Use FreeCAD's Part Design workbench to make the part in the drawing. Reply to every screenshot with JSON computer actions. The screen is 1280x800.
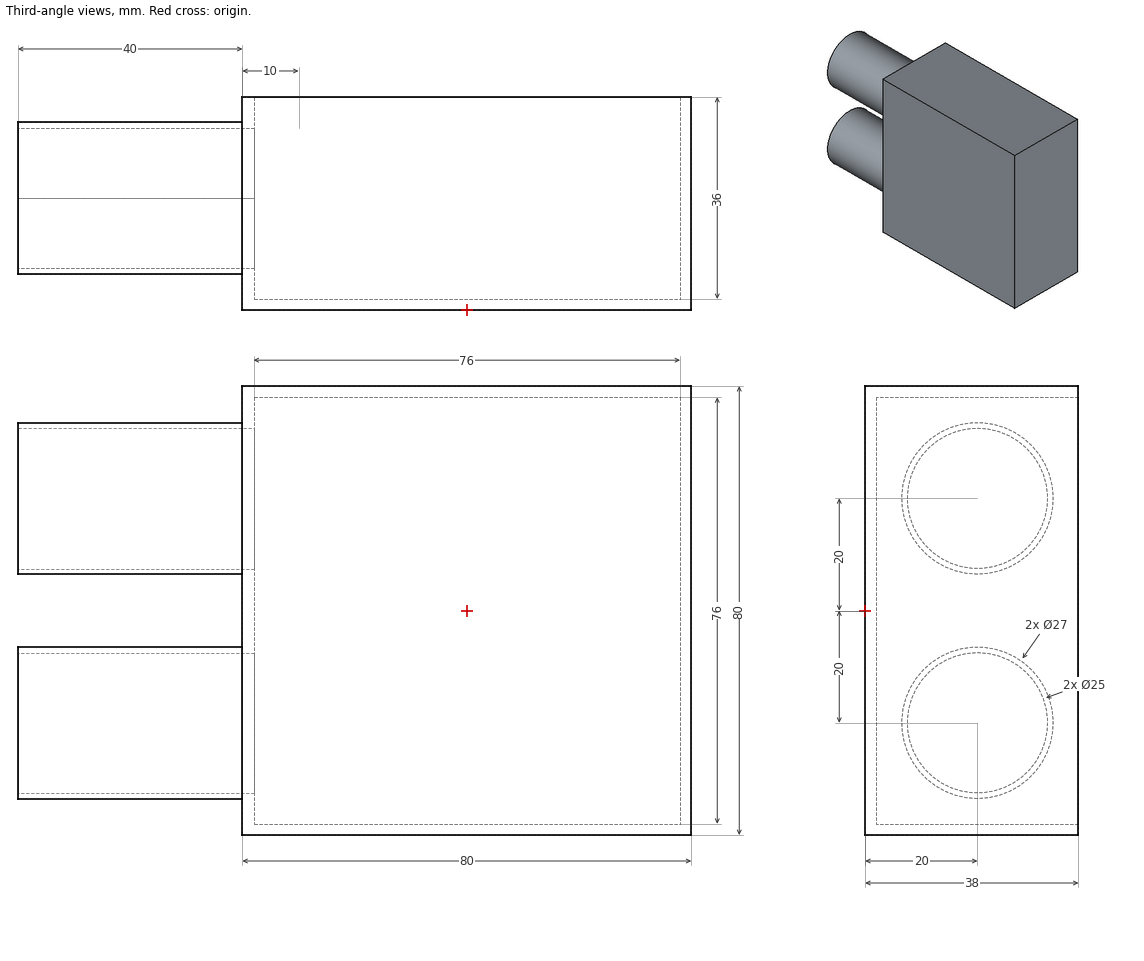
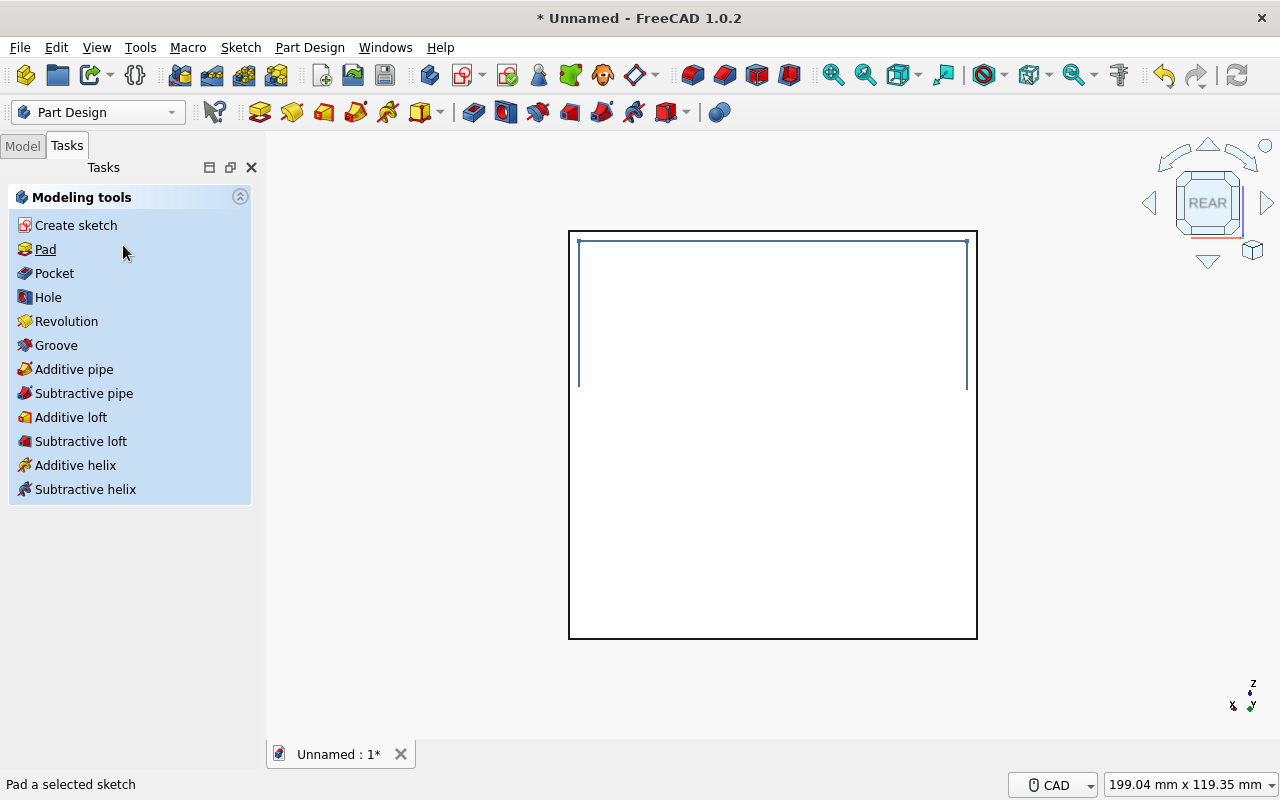
{"action": "left_click", "coordinate": [474, 112]}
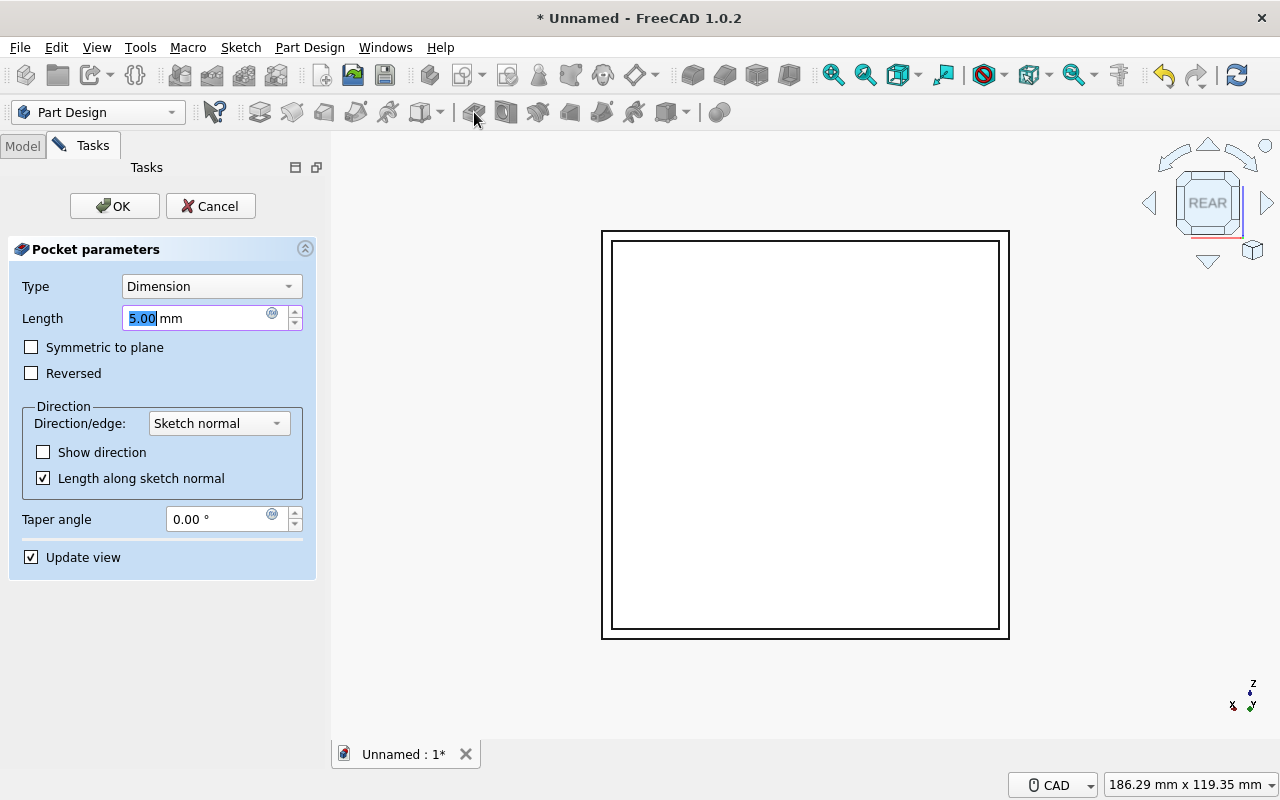
{"action": "type", "text": "36"}
{"action": "key", "text": "Tab"}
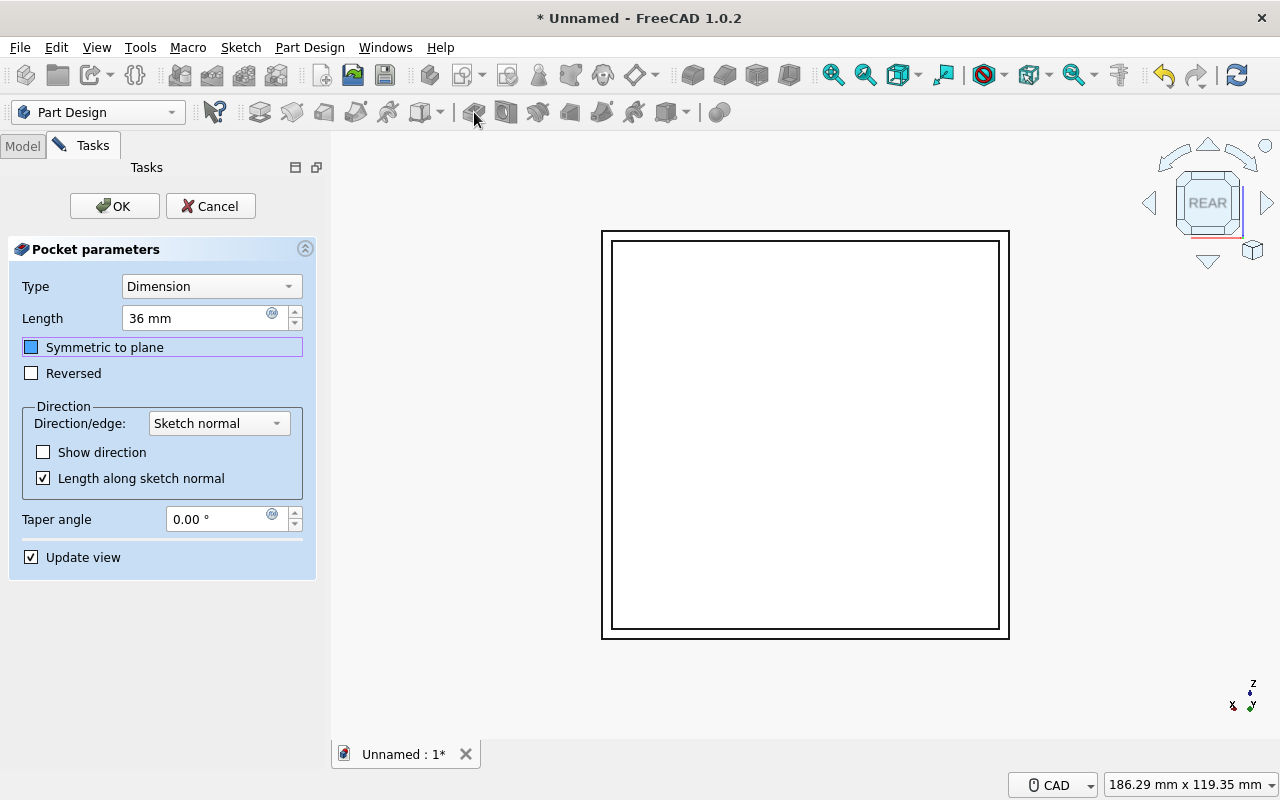
{"action": "left_click", "coordinate": [115, 206]}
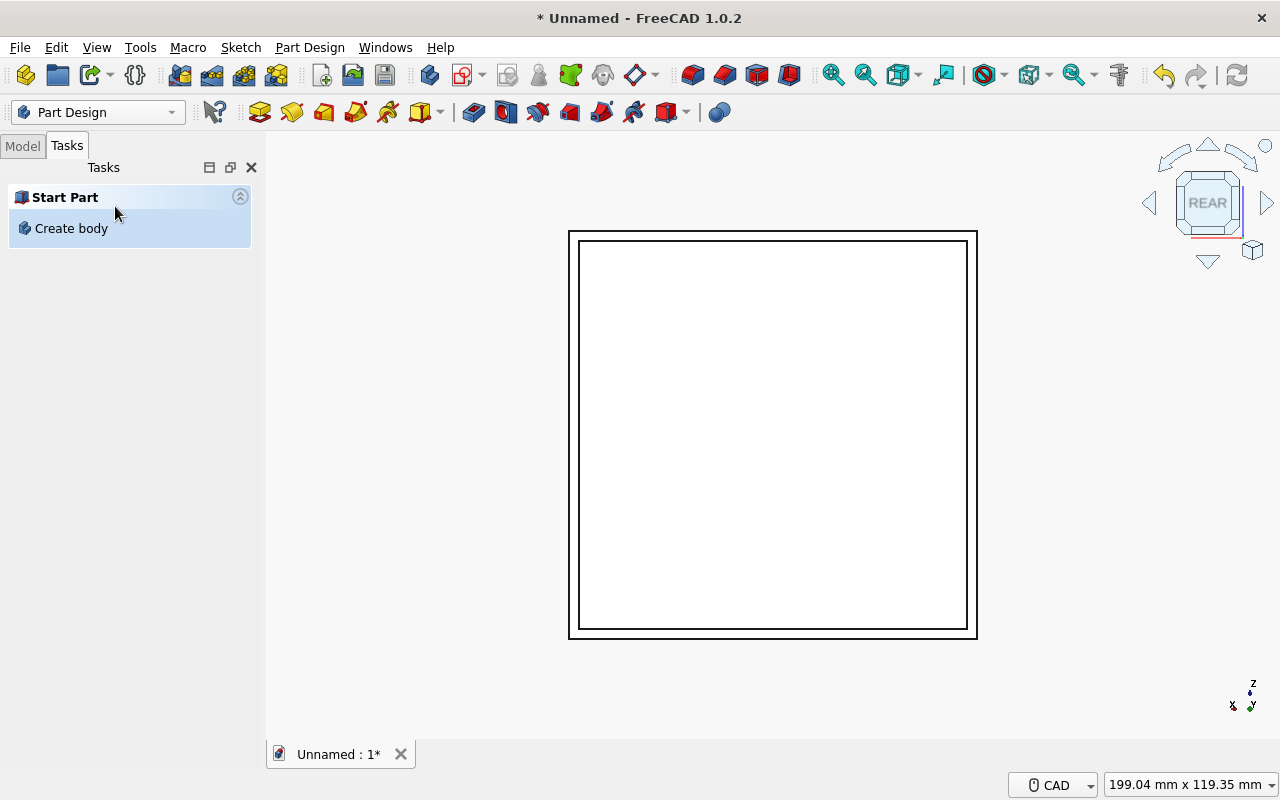
{"action": "key", "text": "6"}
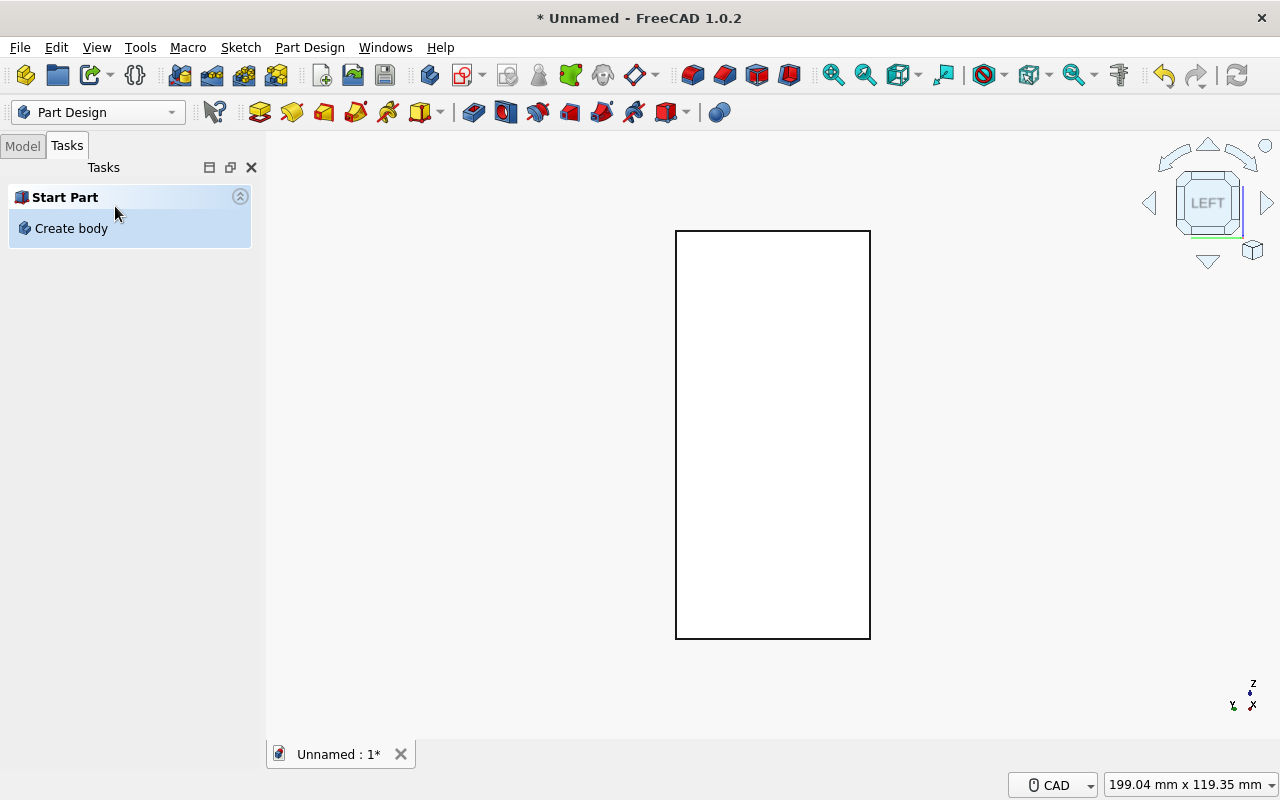
{"action": "left_click", "coordinate": [773, 434]}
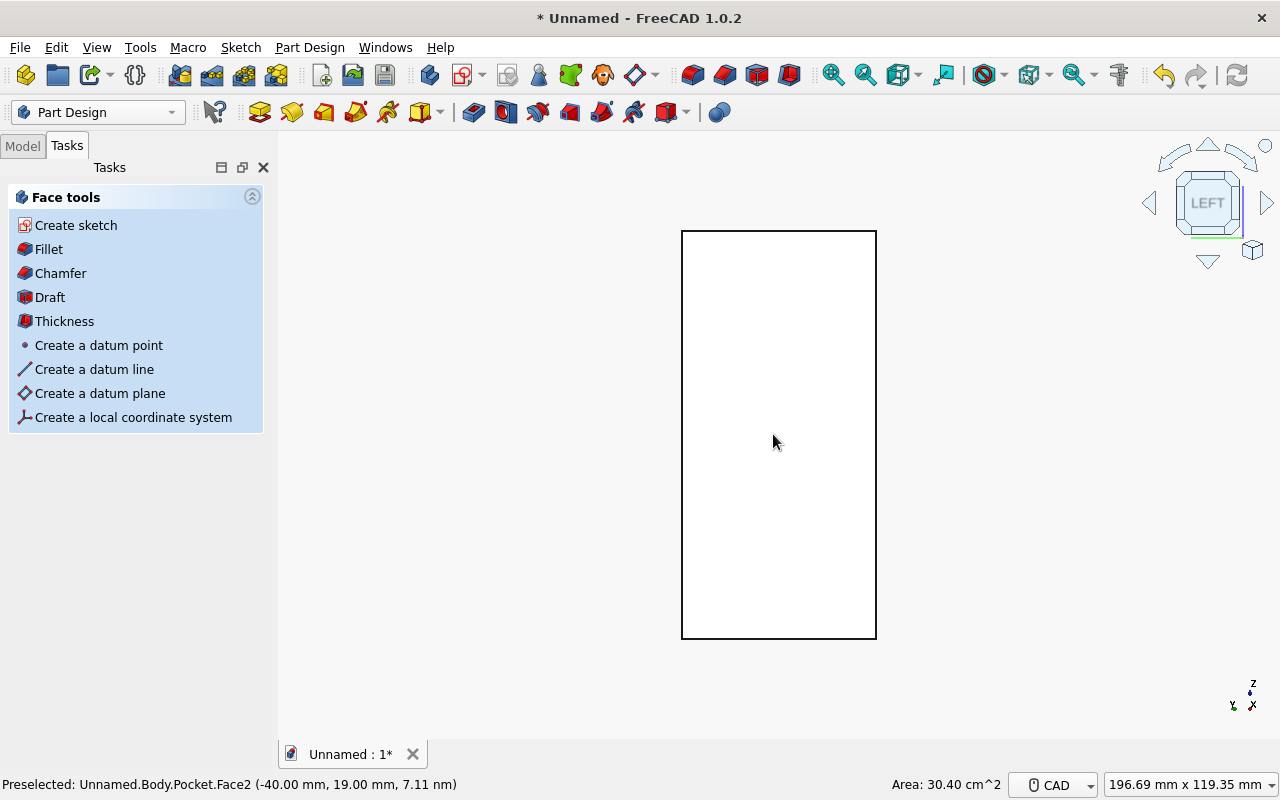
{"action": "left_click", "coordinate": [462, 76]}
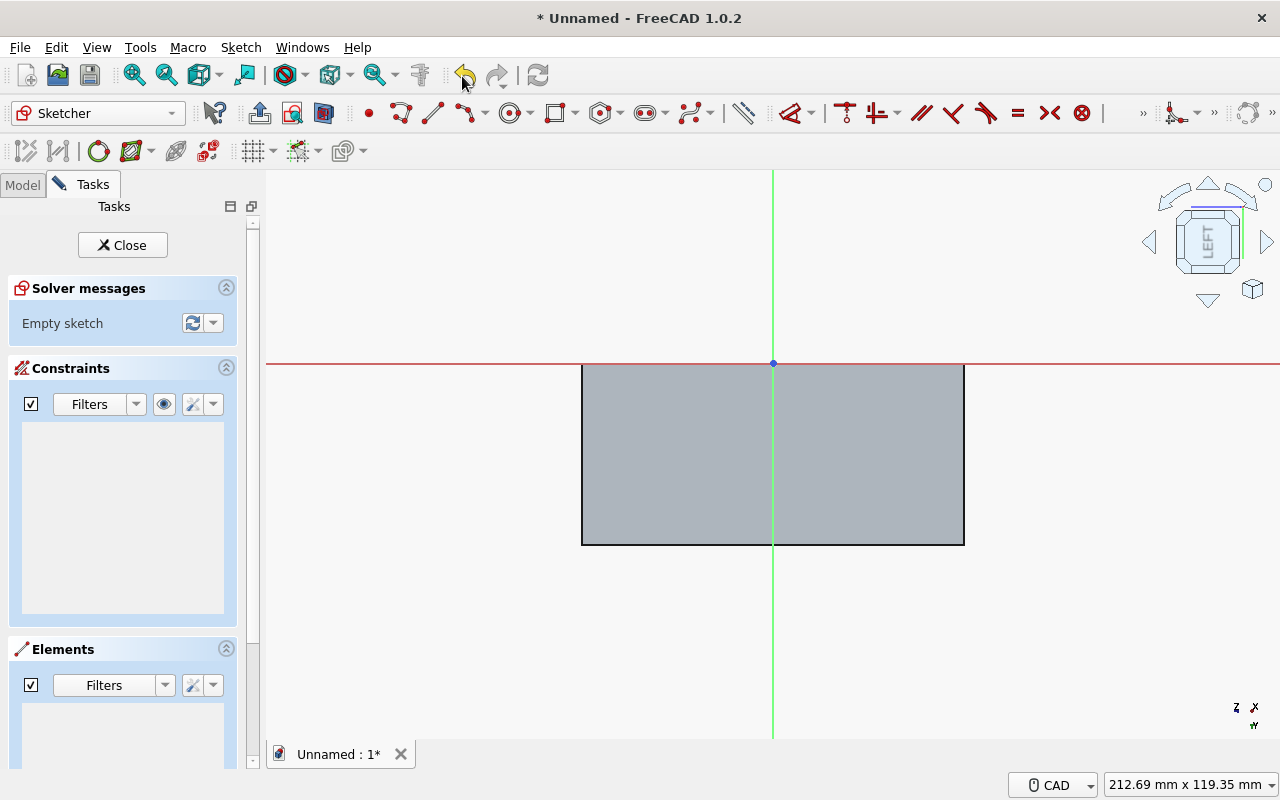
{"action": "scroll", "coordinate": [856, 425], "scroll_direction": "up", "scroll_amount": 3}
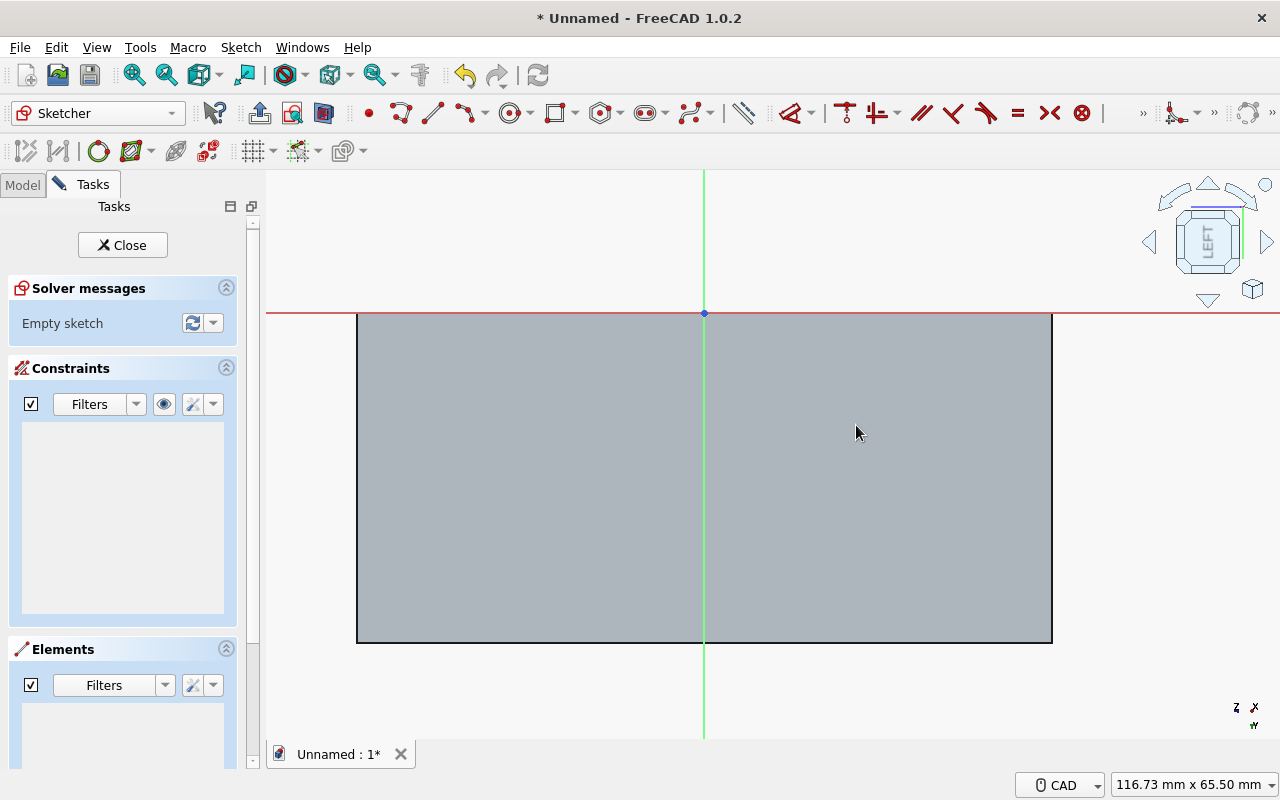
{"action": "key", "text": "g c"}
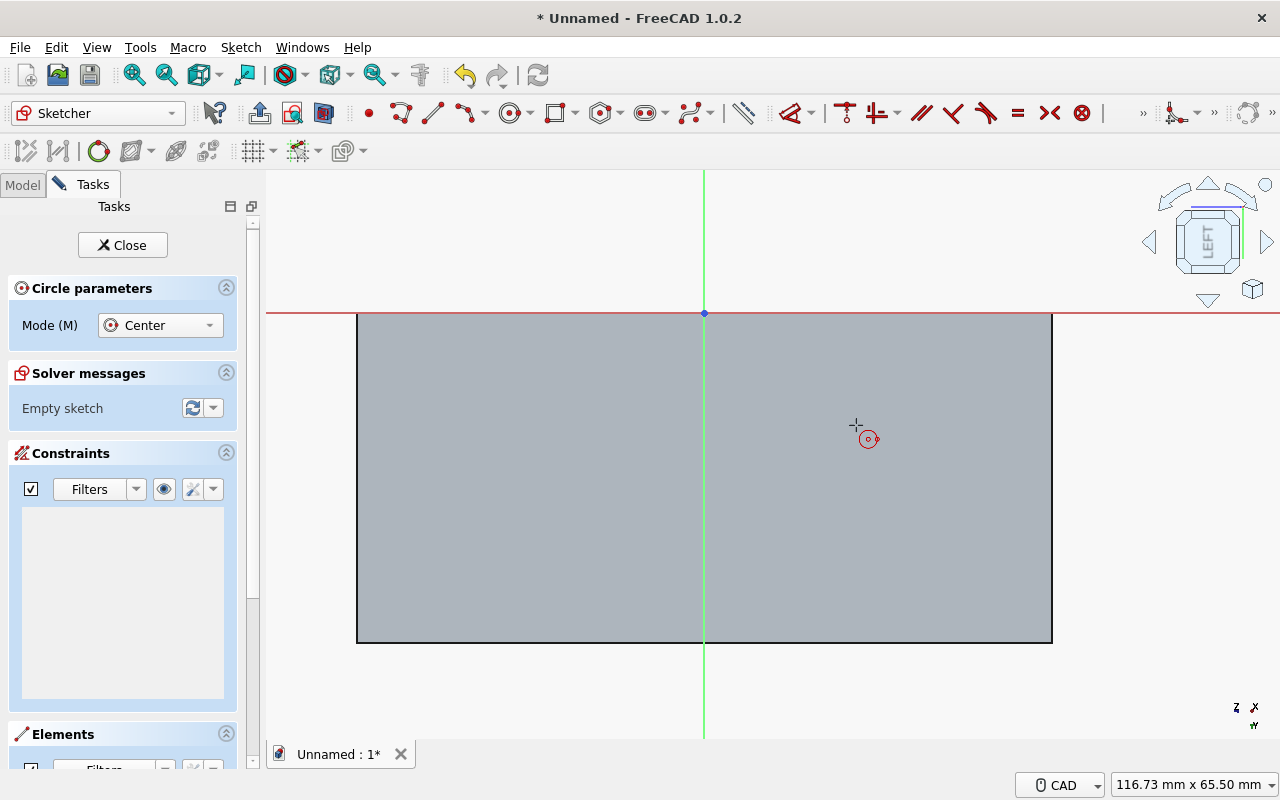
{"action": "left_click", "coordinate": [878, 487]}
{"action": "mouse_move", "coordinate": [955, 410]}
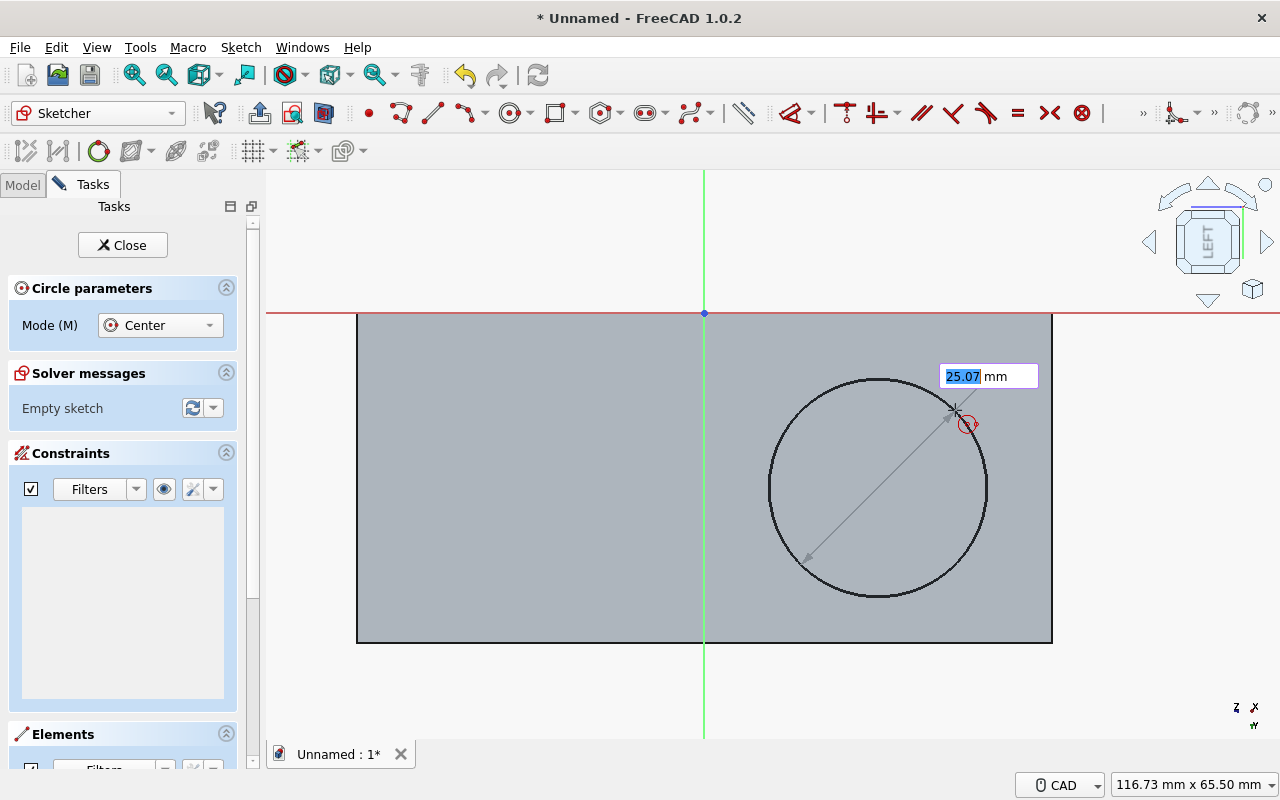
{"action": "type", "text": "25"}
{"action": "key", "text": "Return"}